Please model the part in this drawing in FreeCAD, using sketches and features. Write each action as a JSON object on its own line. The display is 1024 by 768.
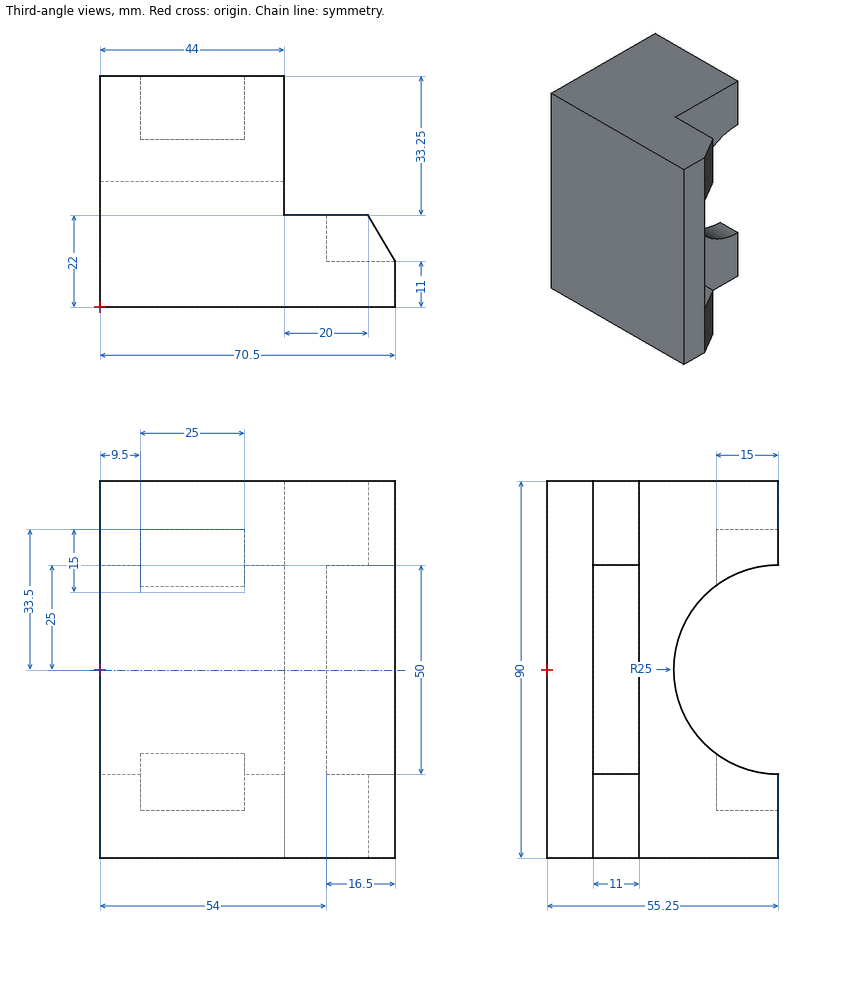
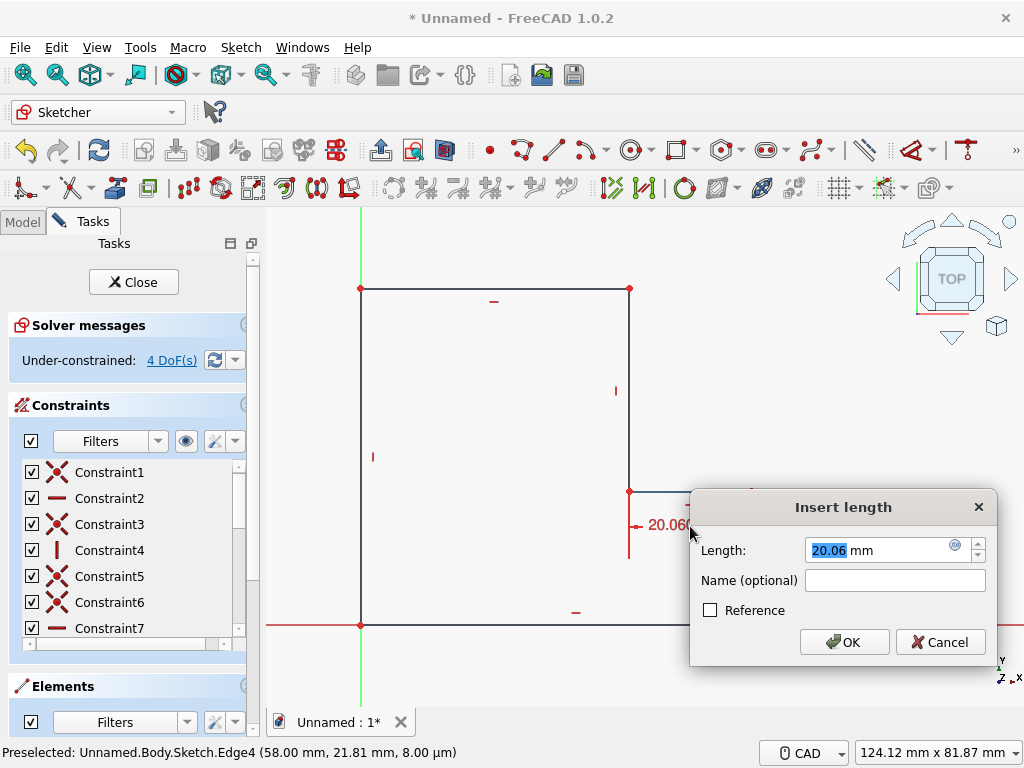
{"action": "type", "text": "20"}
{"action": "key", "text": "Return"}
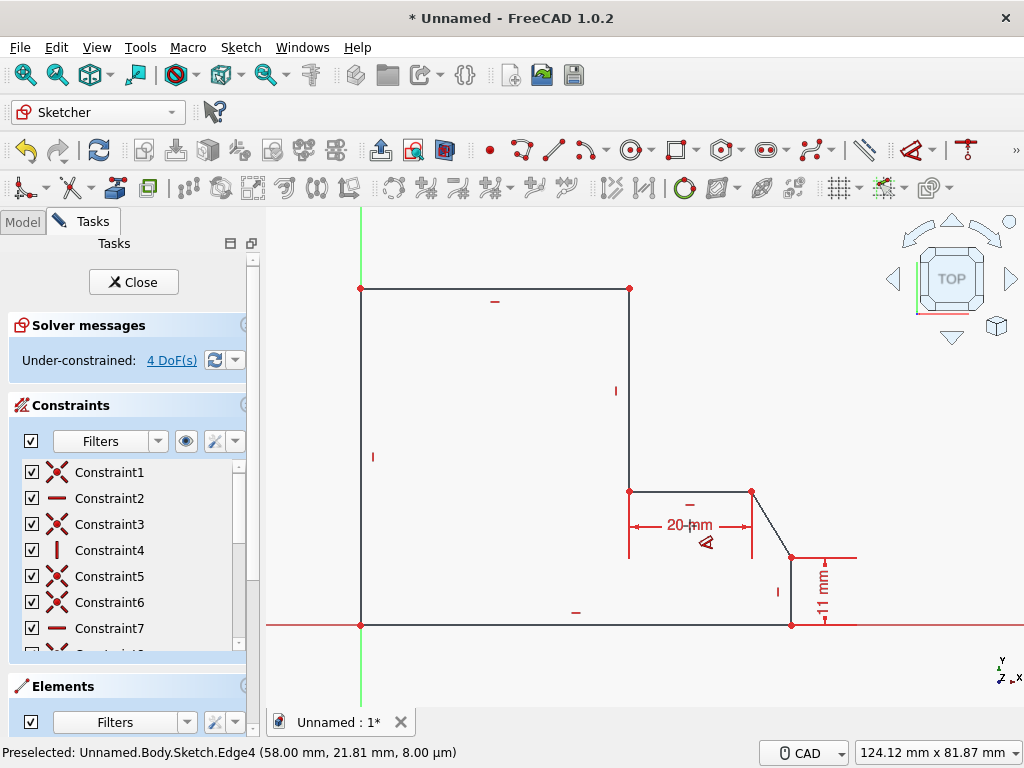
{"action": "left_click", "coordinate": [549, 289]}
{"action": "left_click", "coordinate": [495, 255]}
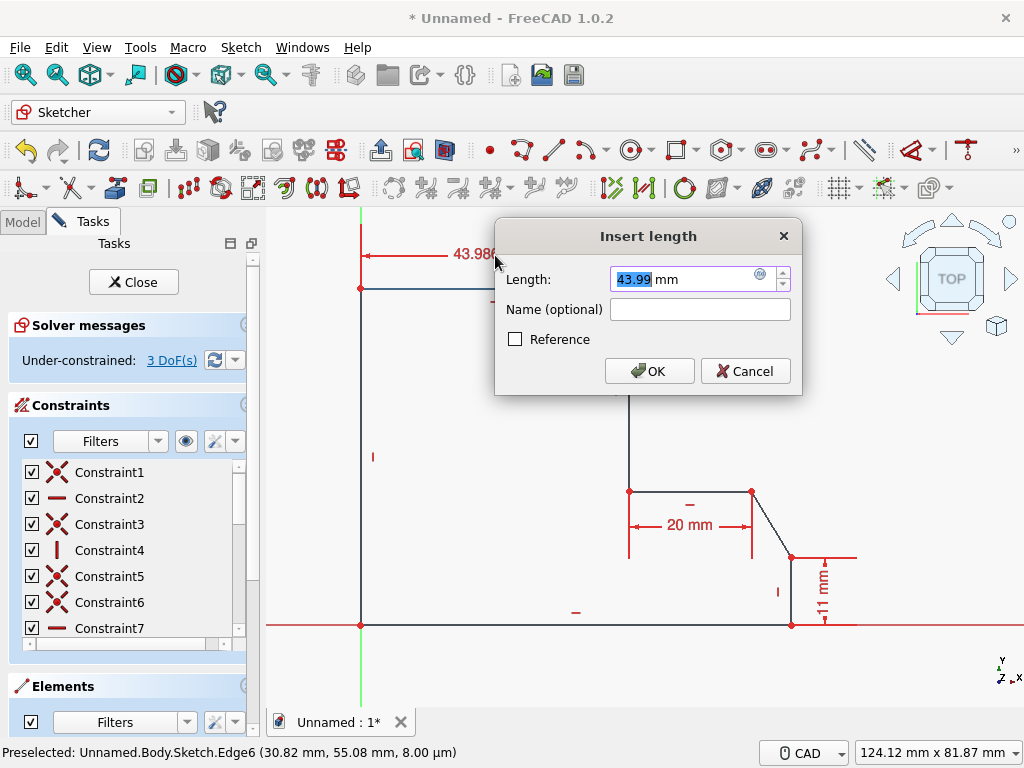
{"action": "type", "text": "44"}
{"action": "key", "text": "Return"}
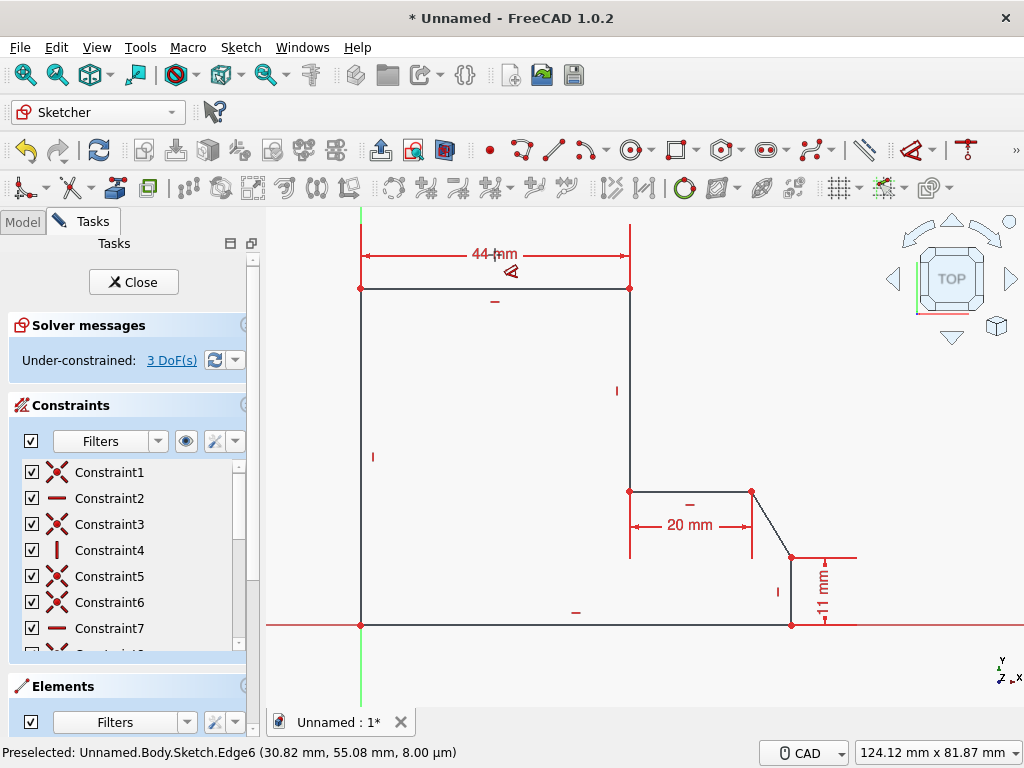
{"action": "left_click", "coordinate": [752, 492]}
{"action": "left_click", "coordinate": [327, 558]}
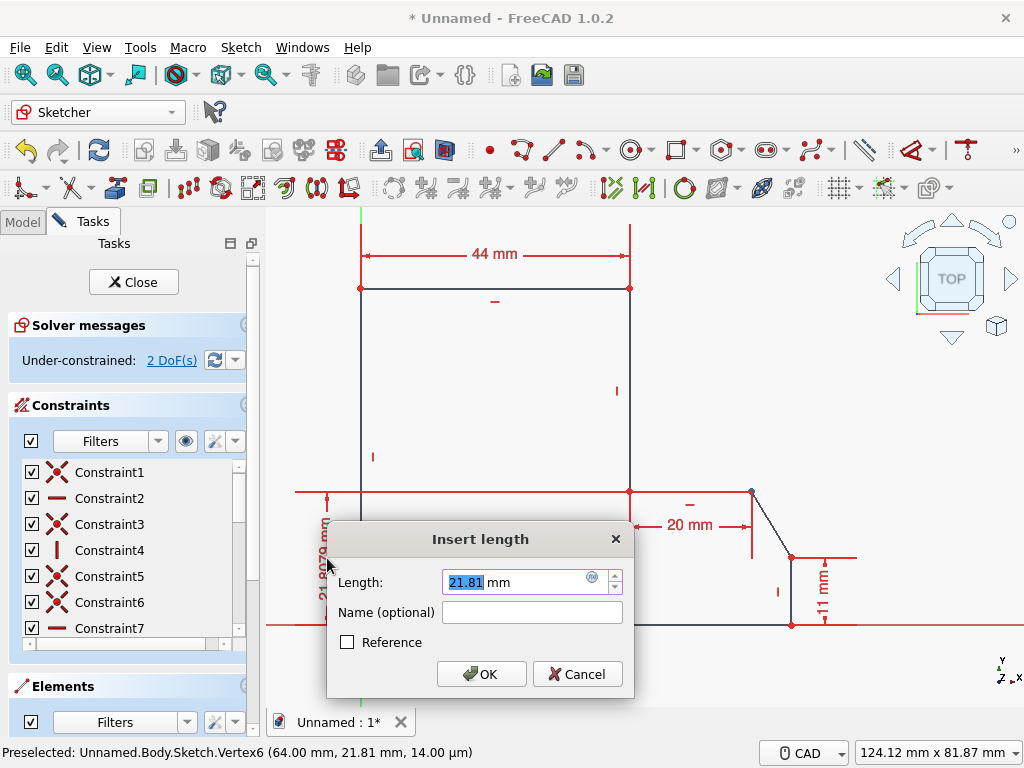
{"action": "type", "text": "22"}
{"action": "key", "text": "Return"}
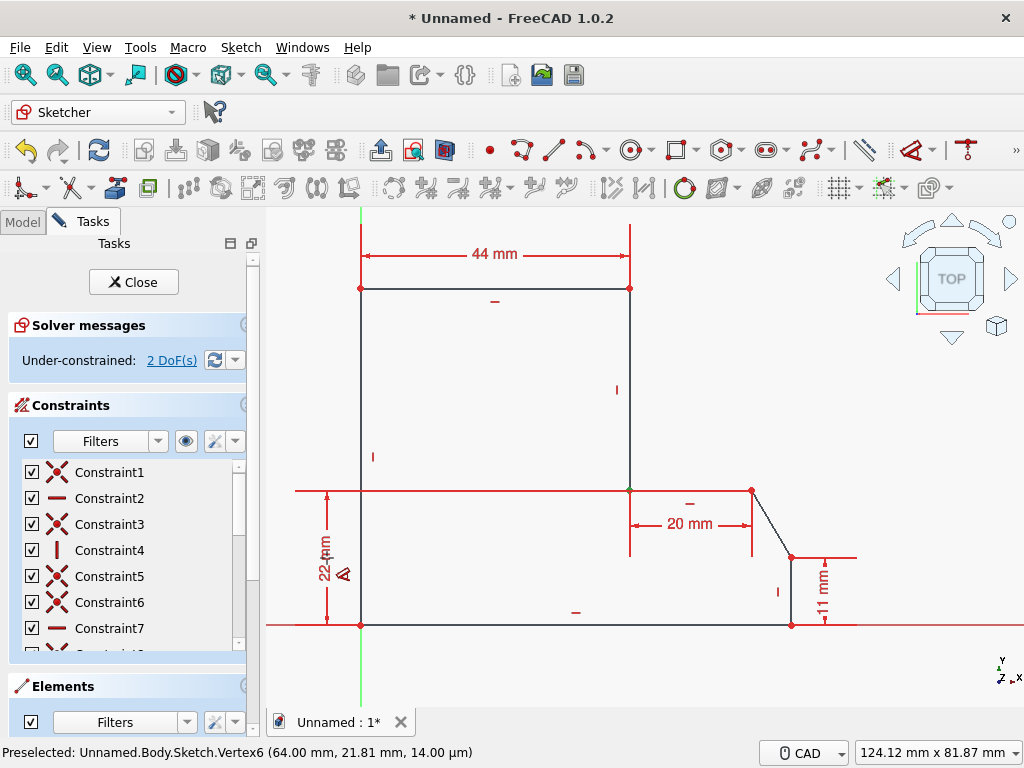
{"action": "left_click", "coordinate": [490, 625]}
{"action": "left_click", "coordinate": [576, 659]}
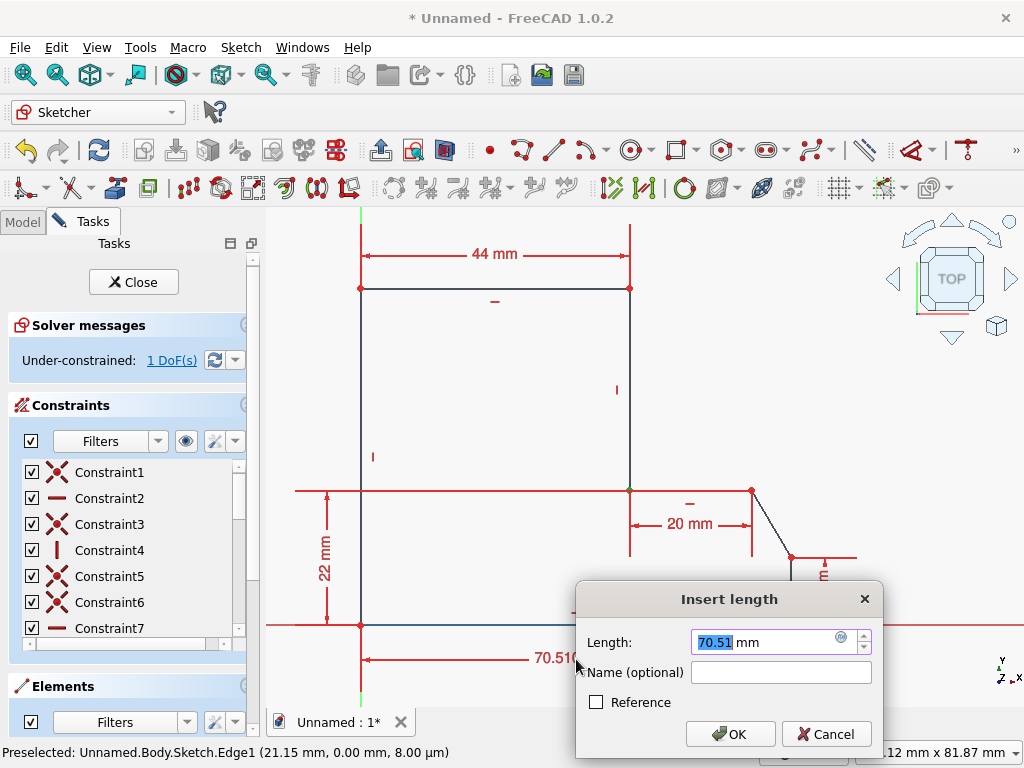
{"action": "type", "text": "70.5"}
{"action": "key", "text": "Return"}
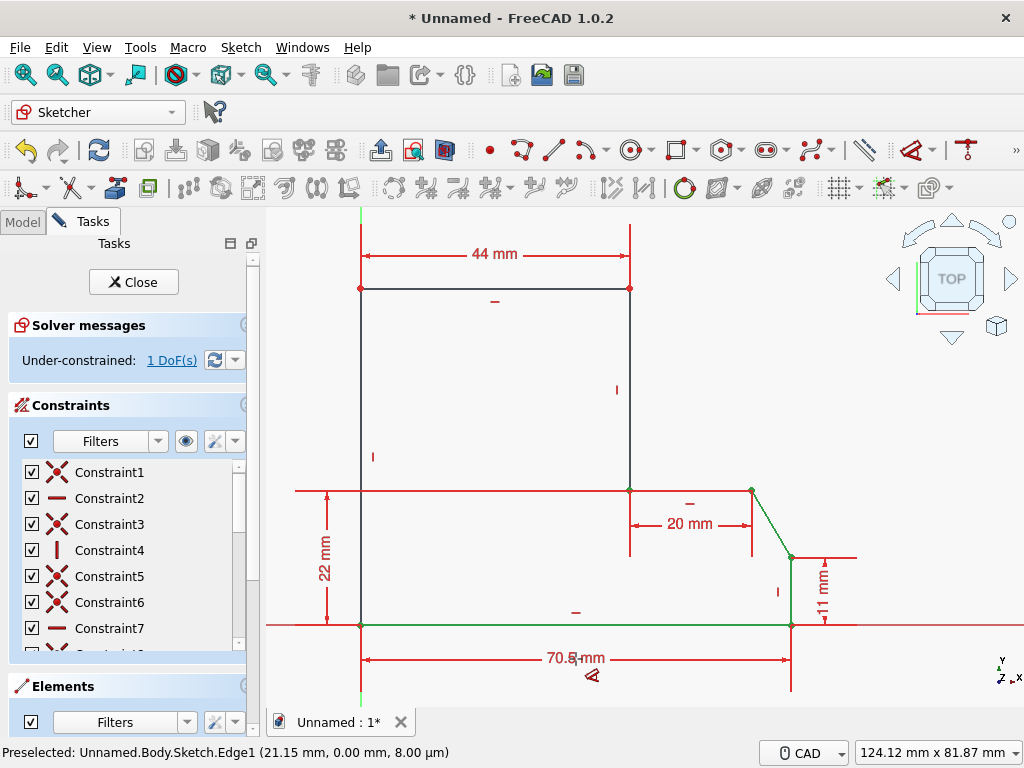
{"action": "left_click", "coordinate": [630, 430]}
{"action": "left_click", "coordinate": [664, 390]}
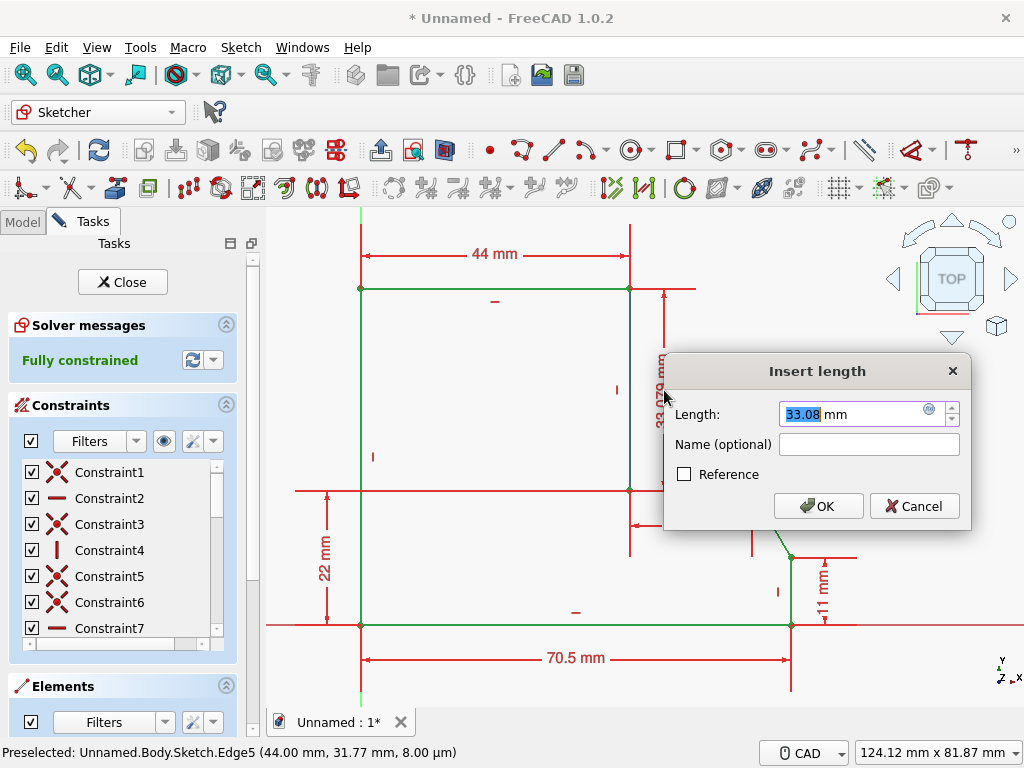
{"action": "type", "text": "33.25"}
{"action": "key", "text": "Return"}
{"action": "key", "text": "Escape"}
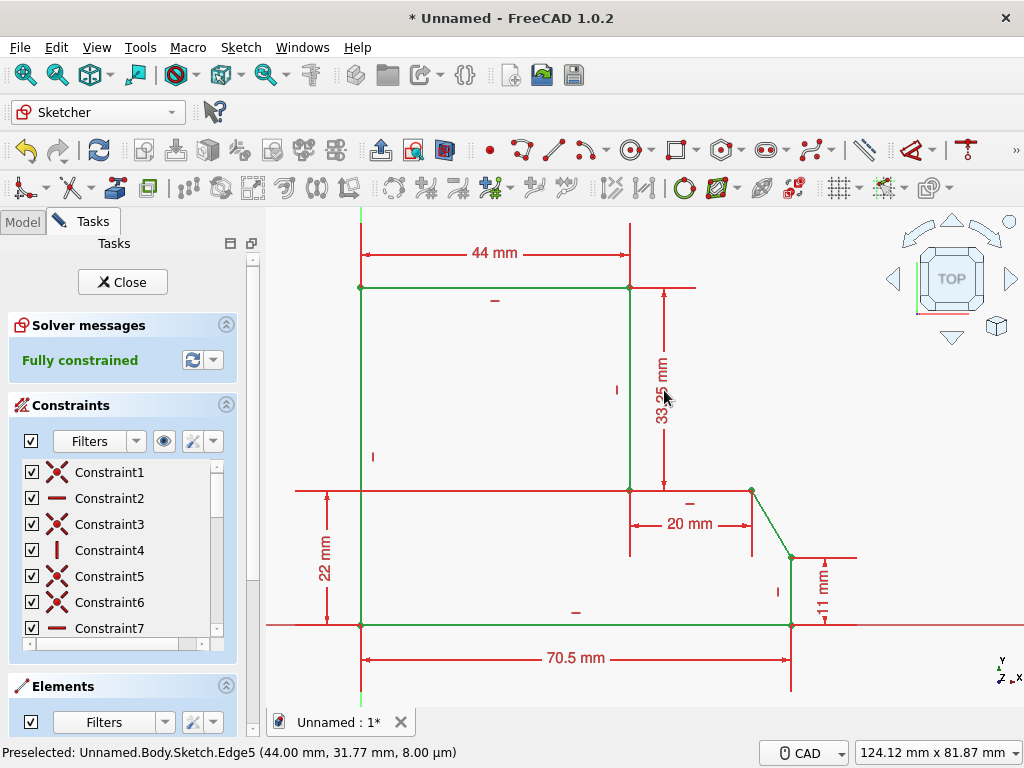
{"action": "left_click", "coordinate": [123, 282]}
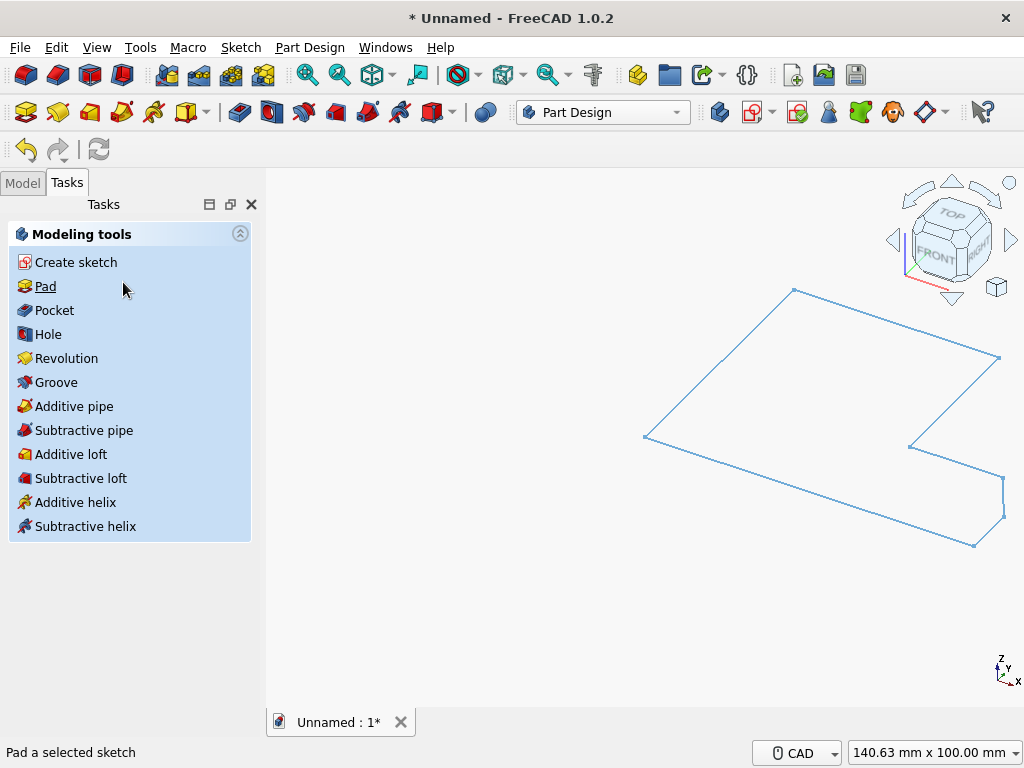
{"action": "left_click", "coordinate": [26, 112]}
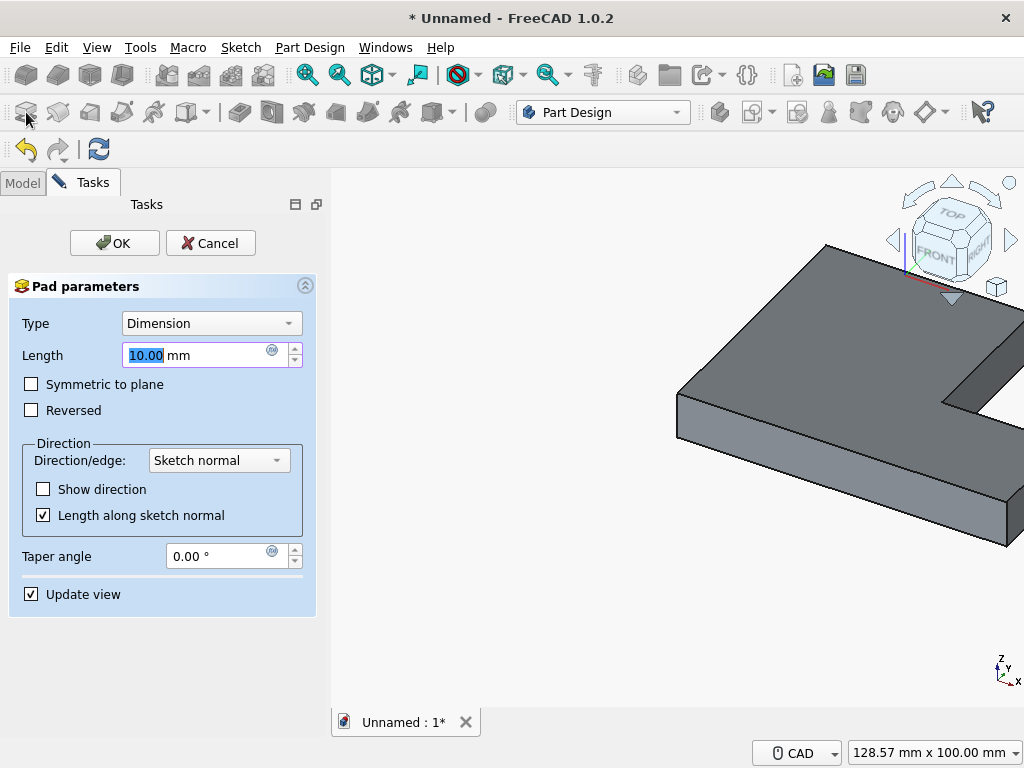
{"action": "type", "text": "90"}
{"action": "key", "text": "Tab"}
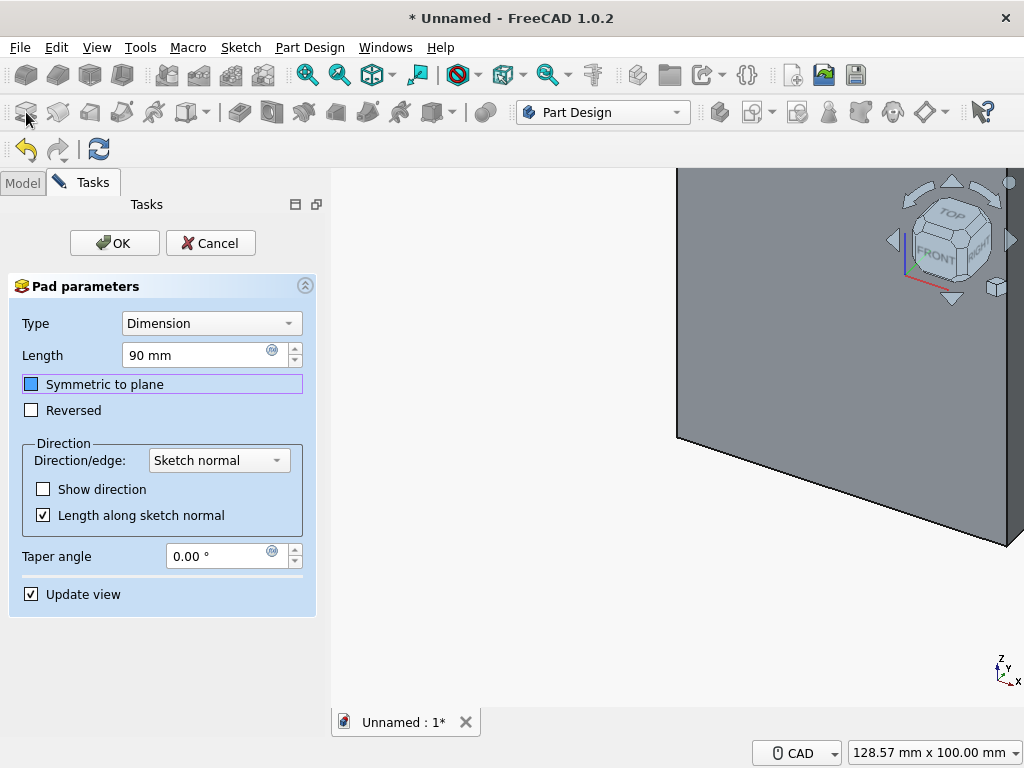
{"action": "left_click", "coordinate": [30, 384]}